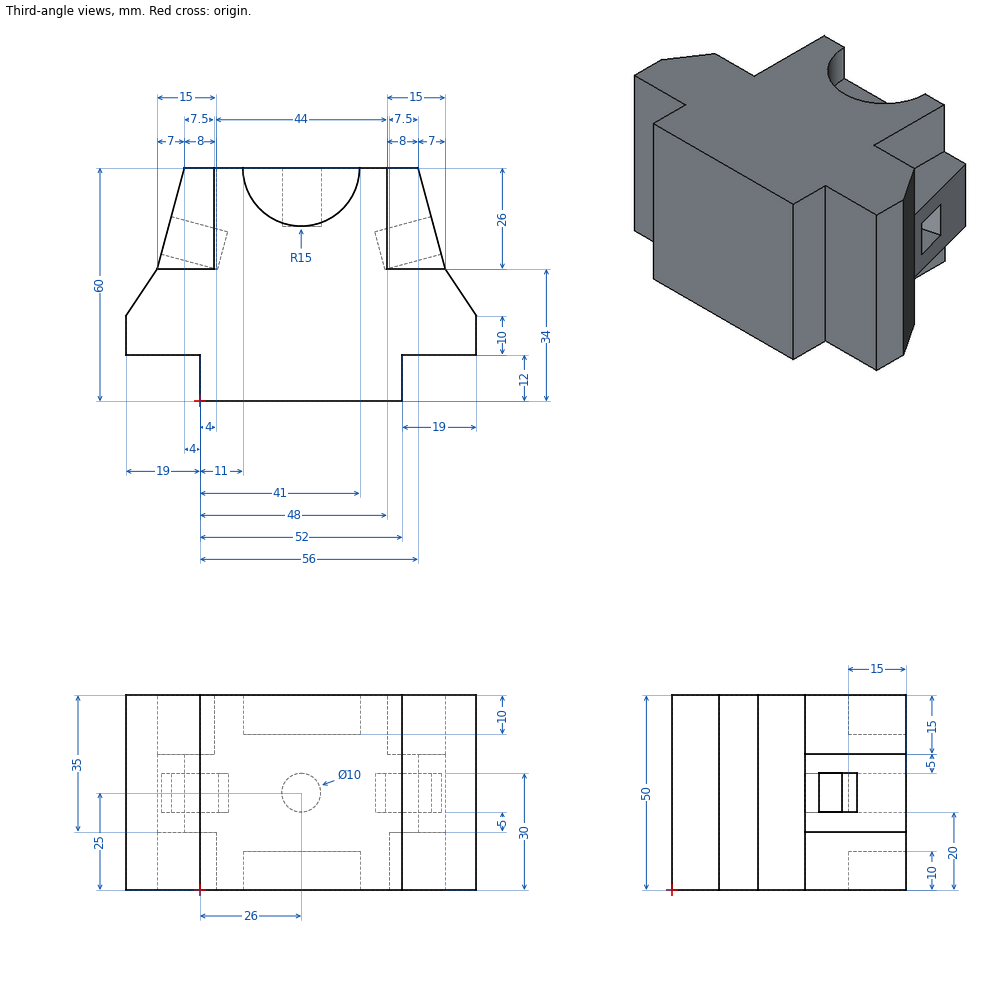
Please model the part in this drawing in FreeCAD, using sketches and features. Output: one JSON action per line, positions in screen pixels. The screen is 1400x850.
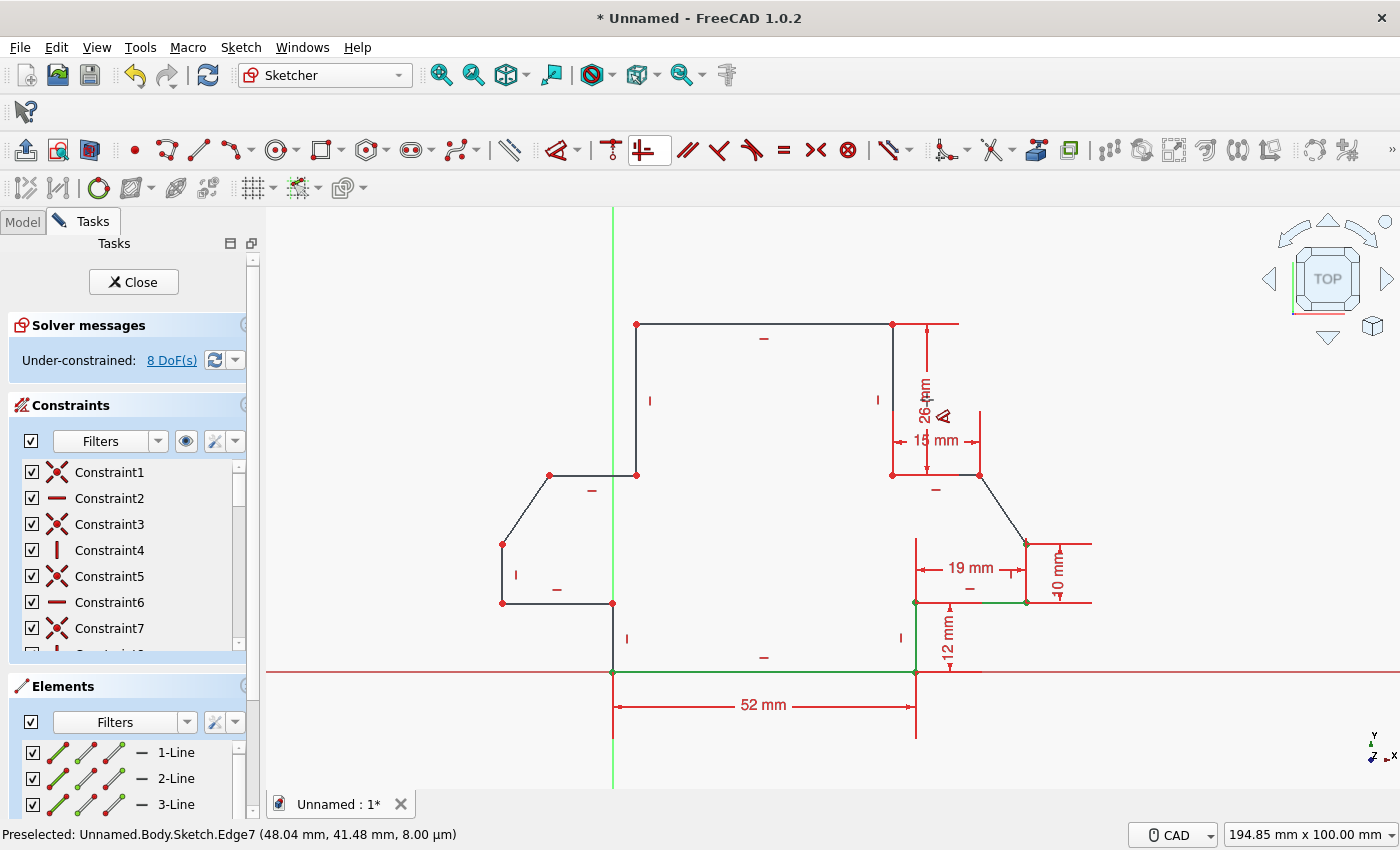
{"action": "left_click", "coordinate": [816, 324]}
{"action": "left_click", "coordinate": [764, 290]}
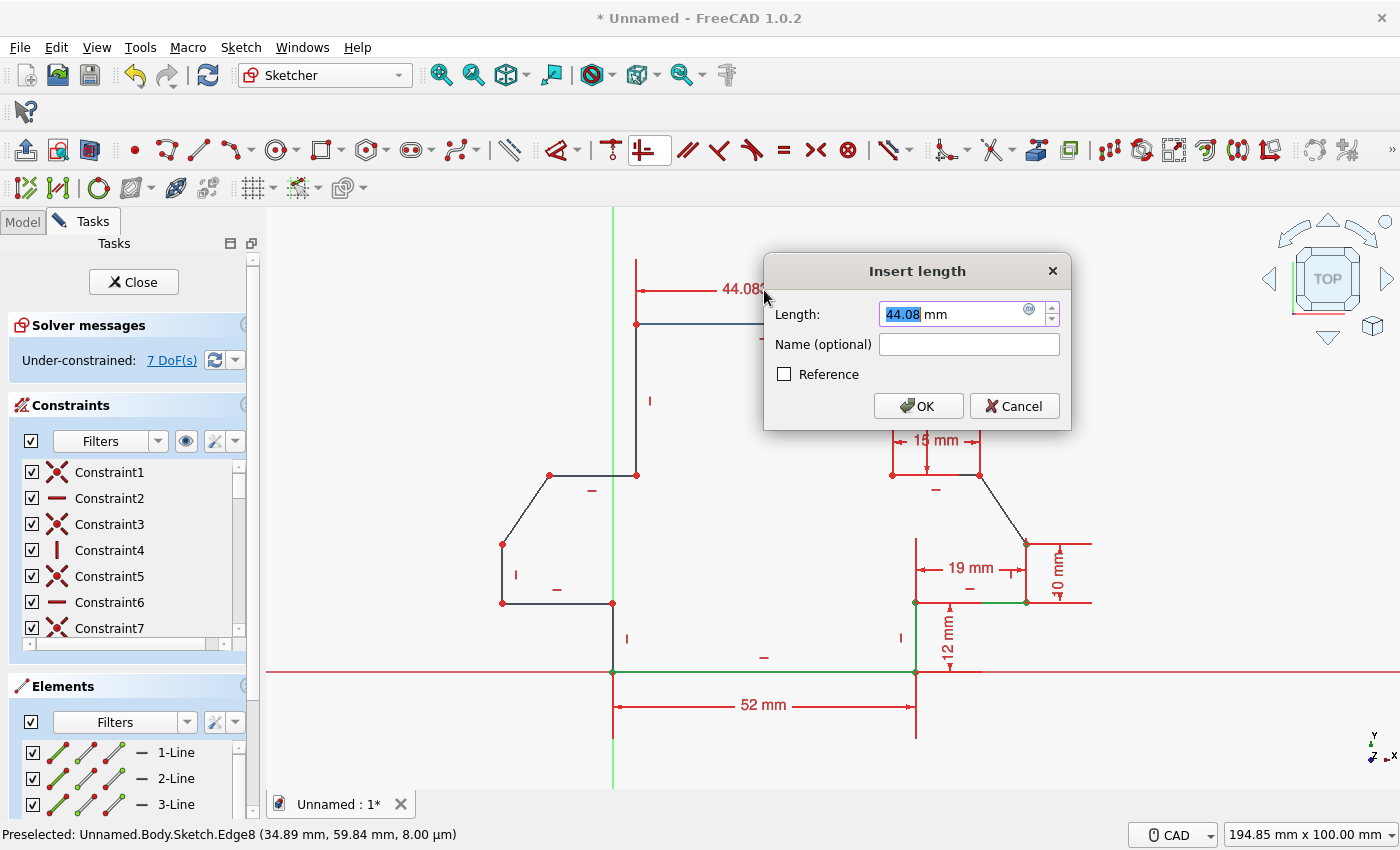
{"action": "type", "text": "44"}
{"action": "key", "text": "Return"}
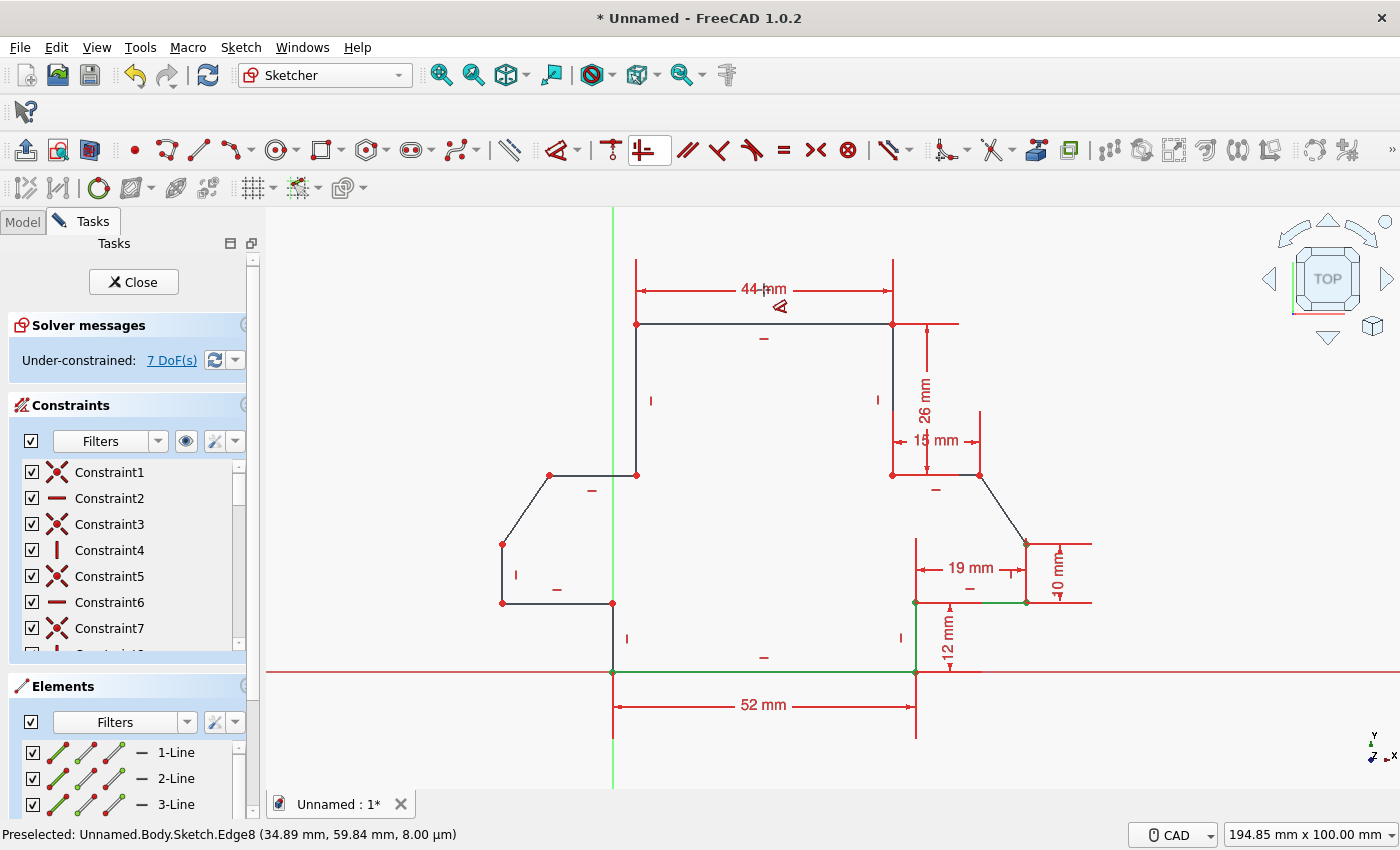
{"action": "left_click", "coordinate": [636, 370]}
{"action": "left_click", "coordinate": [670, 400]}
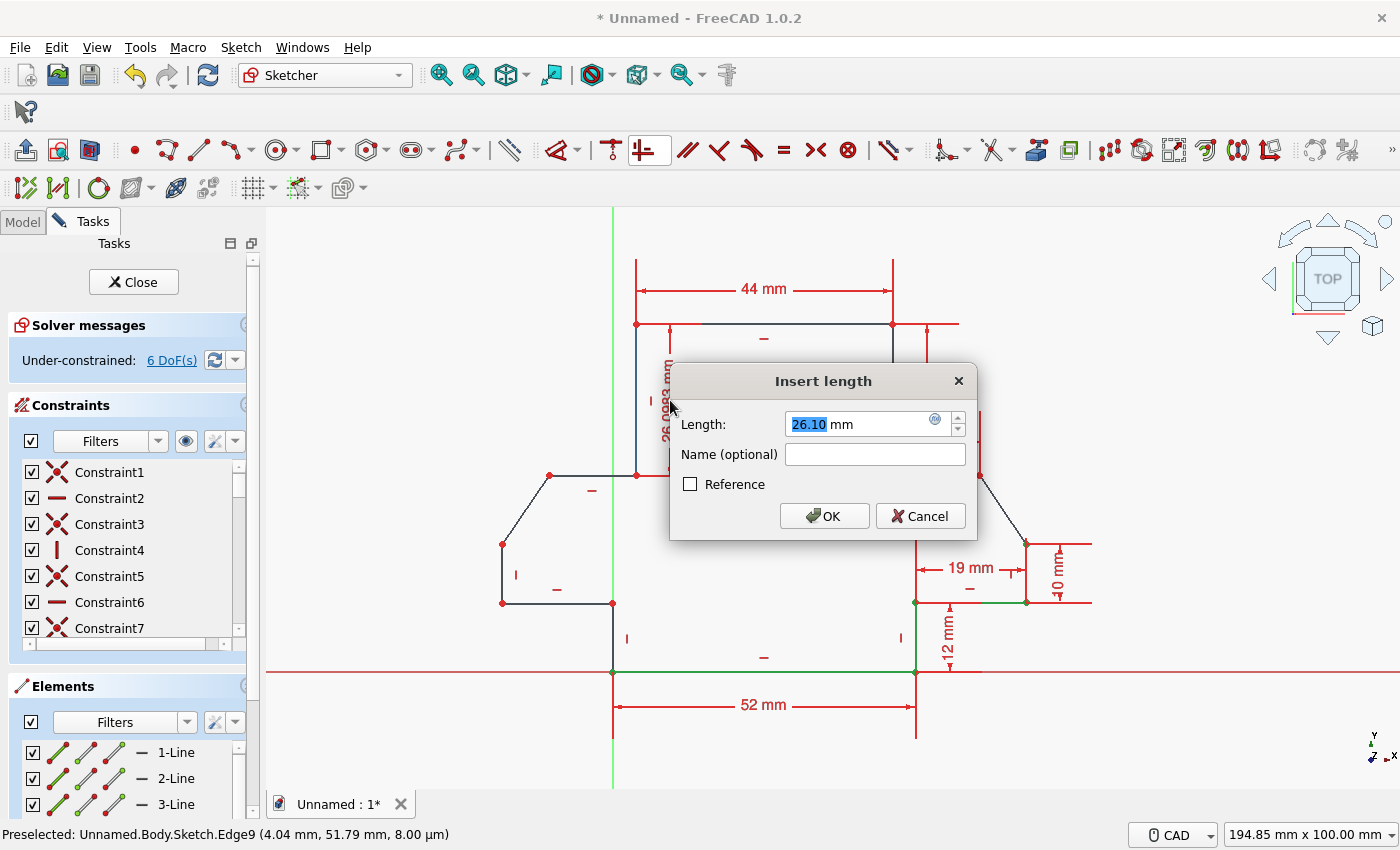
{"action": "type", "text": "26"}
{"action": "key", "text": "Return"}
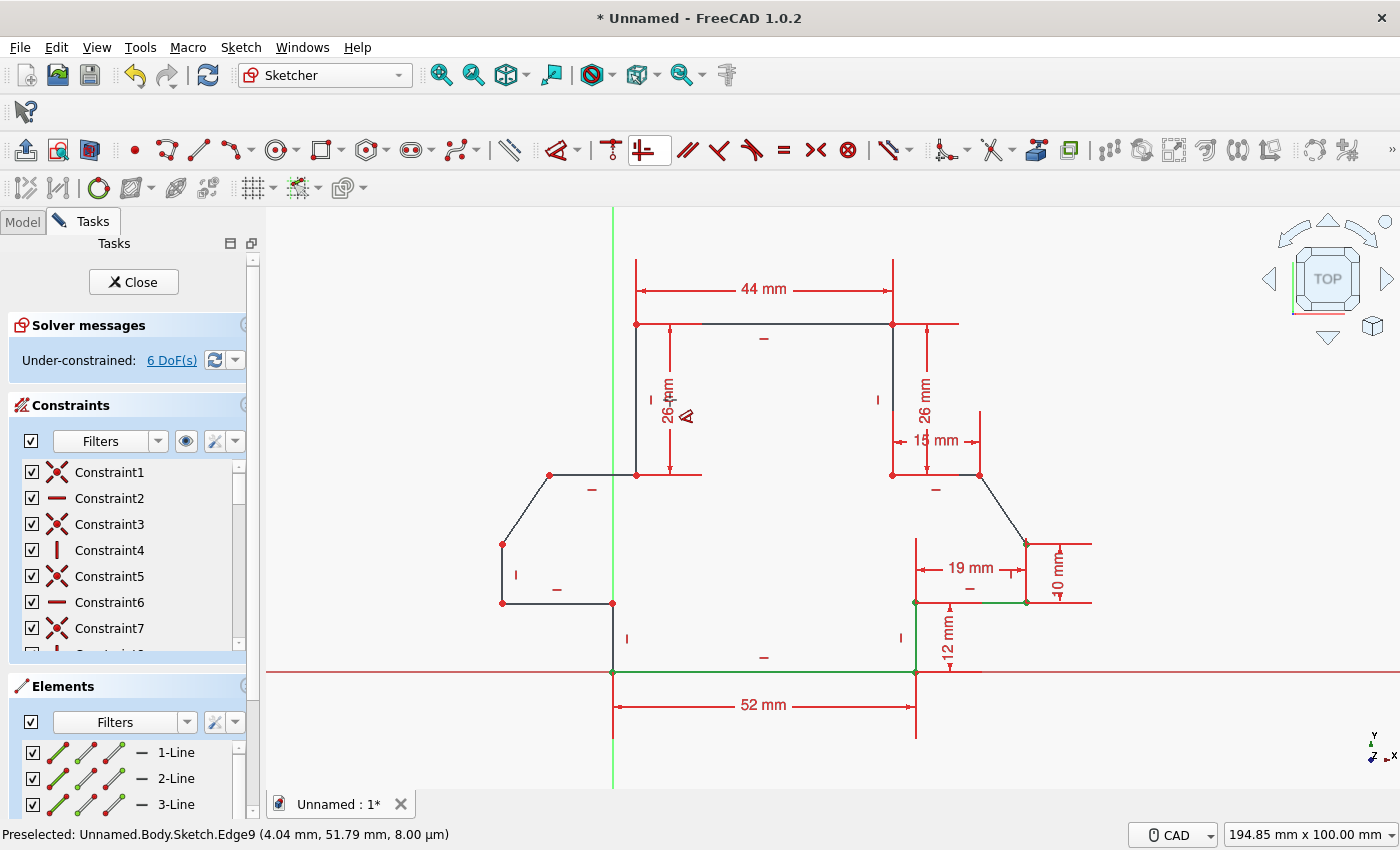
{"action": "left_click", "coordinate": [610, 475]}
{"action": "left_click", "coordinate": [593, 441]}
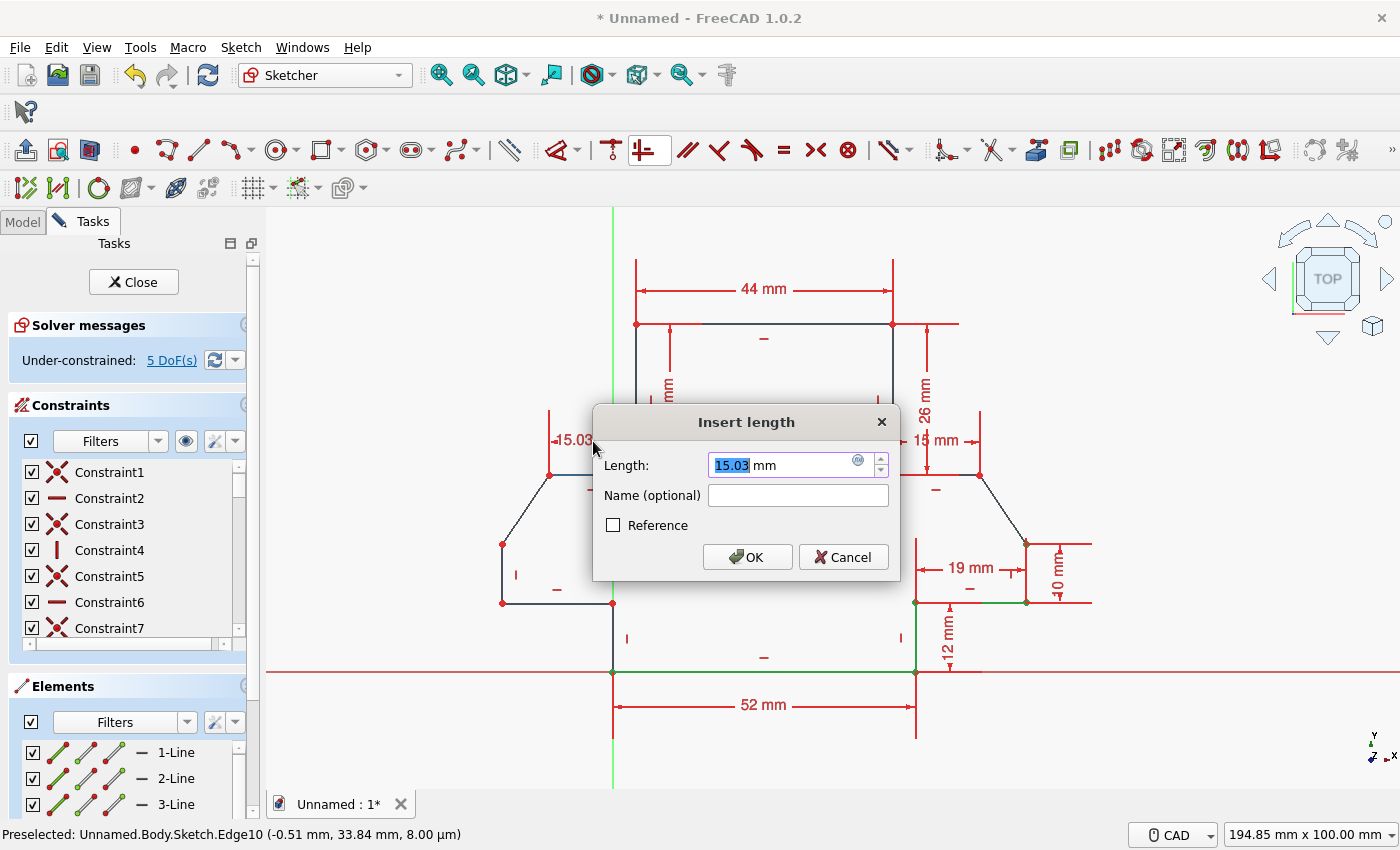
{"action": "type", "text": "15"}
{"action": "key", "text": "Return"}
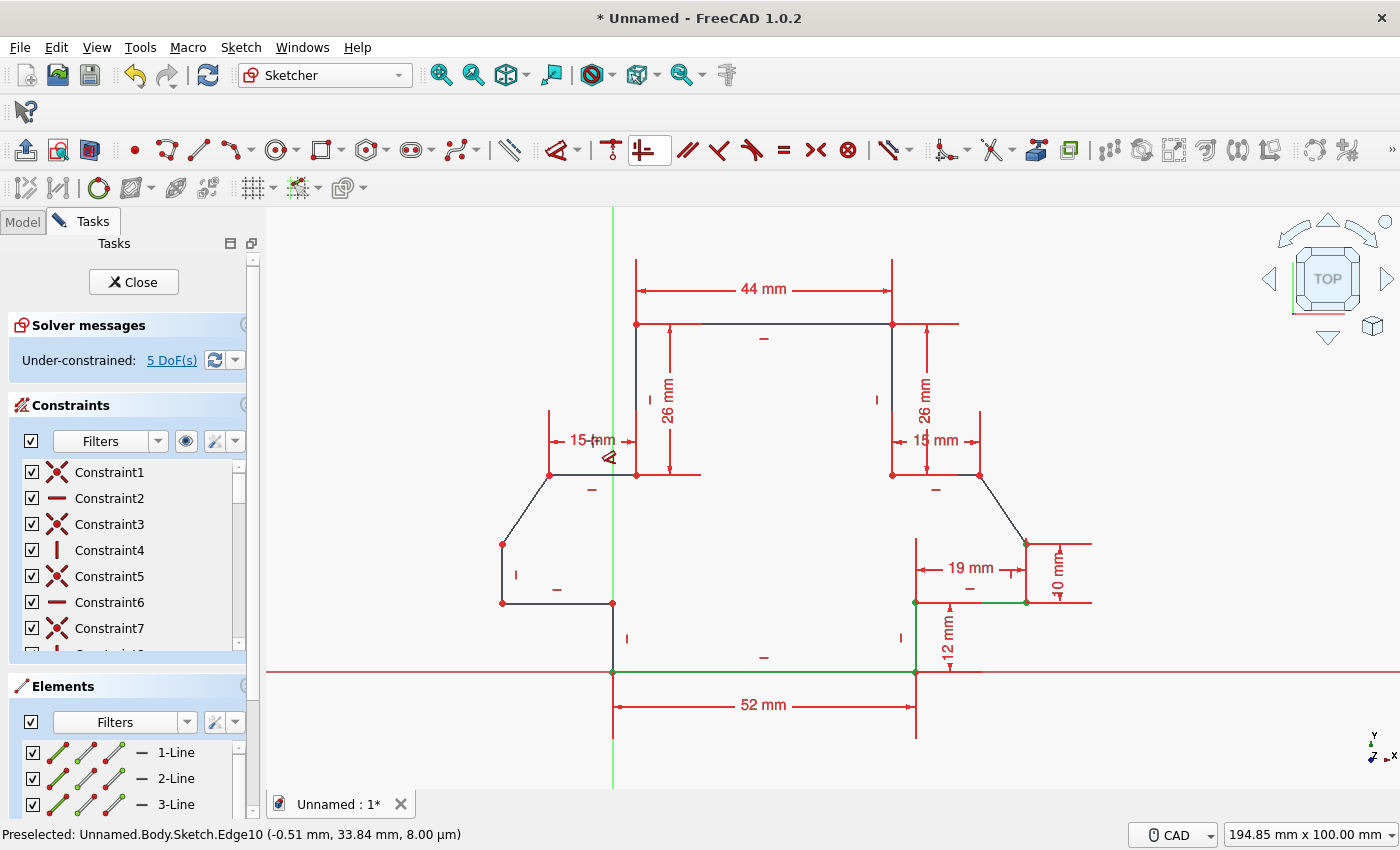
{"action": "left_click", "coordinate": [502, 563]}
{"action": "left_click", "coordinate": [468, 574]}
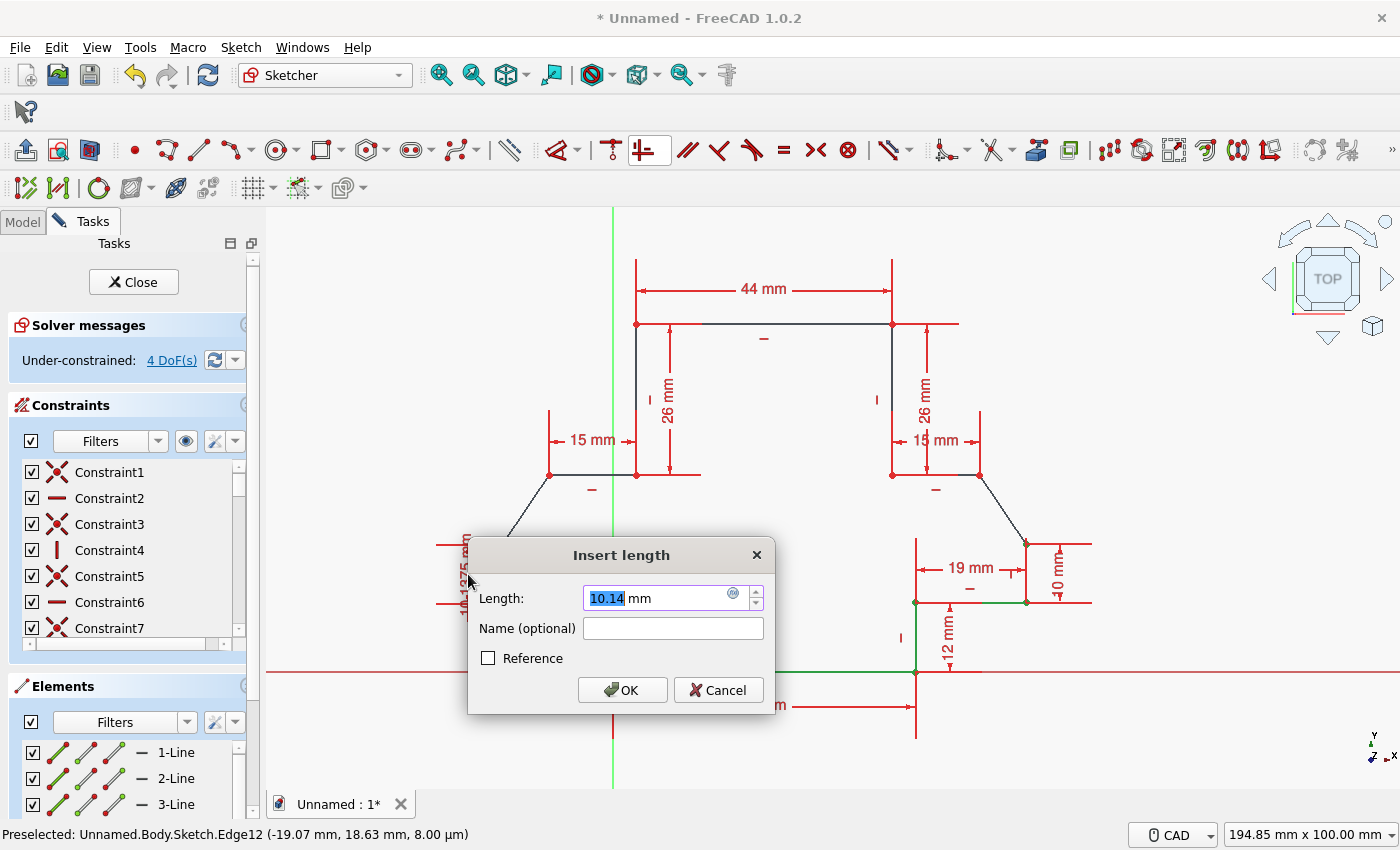
{"action": "type", "text": "10"}
{"action": "key", "text": "Return"}